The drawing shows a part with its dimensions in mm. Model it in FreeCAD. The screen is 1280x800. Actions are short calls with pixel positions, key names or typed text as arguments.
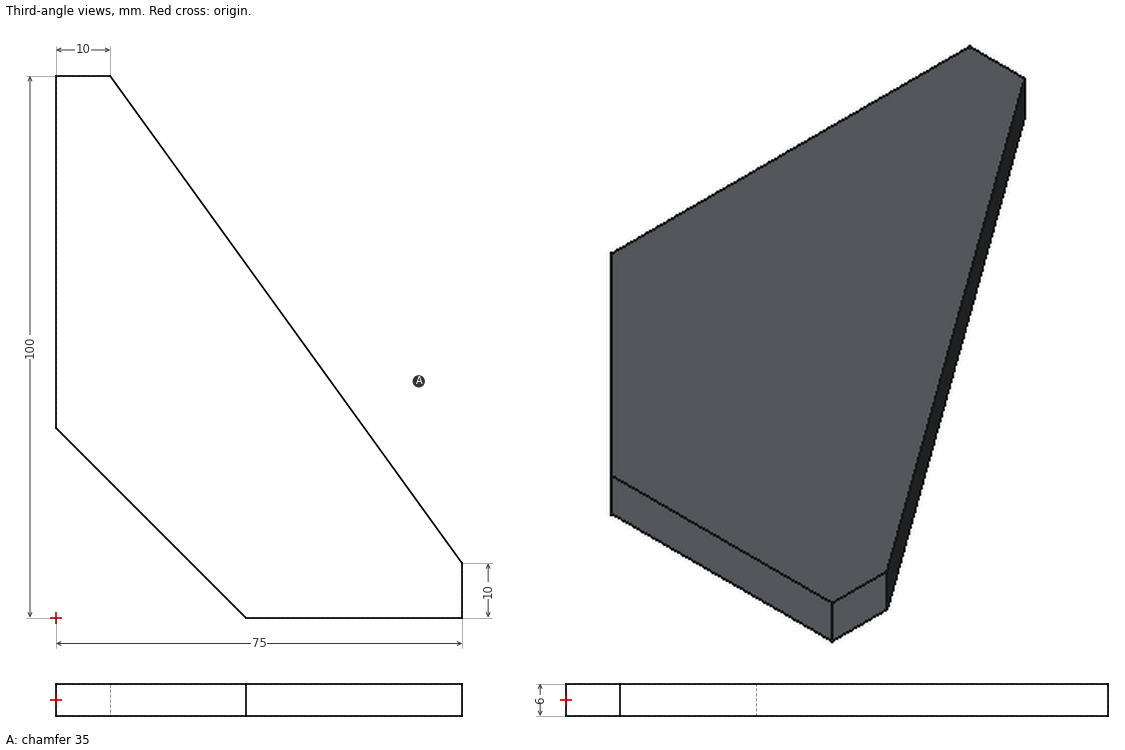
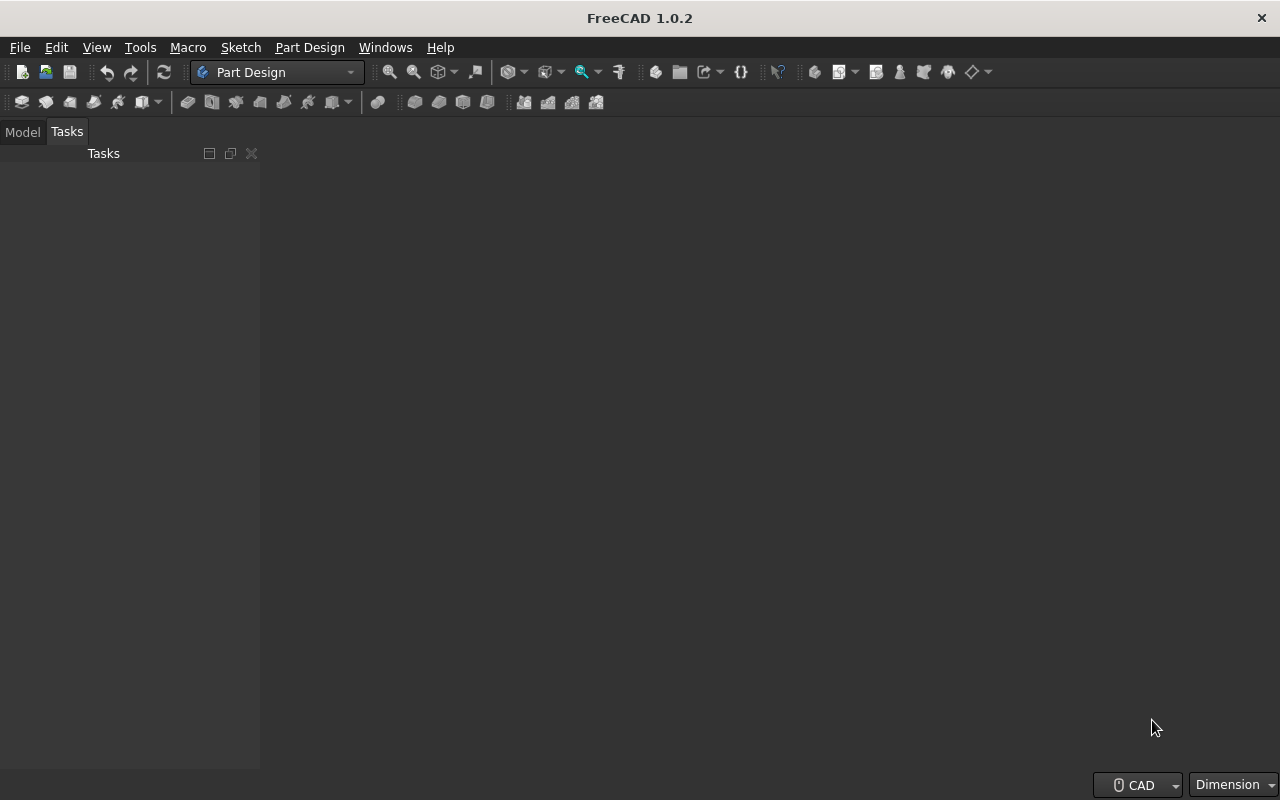
click(22, 72)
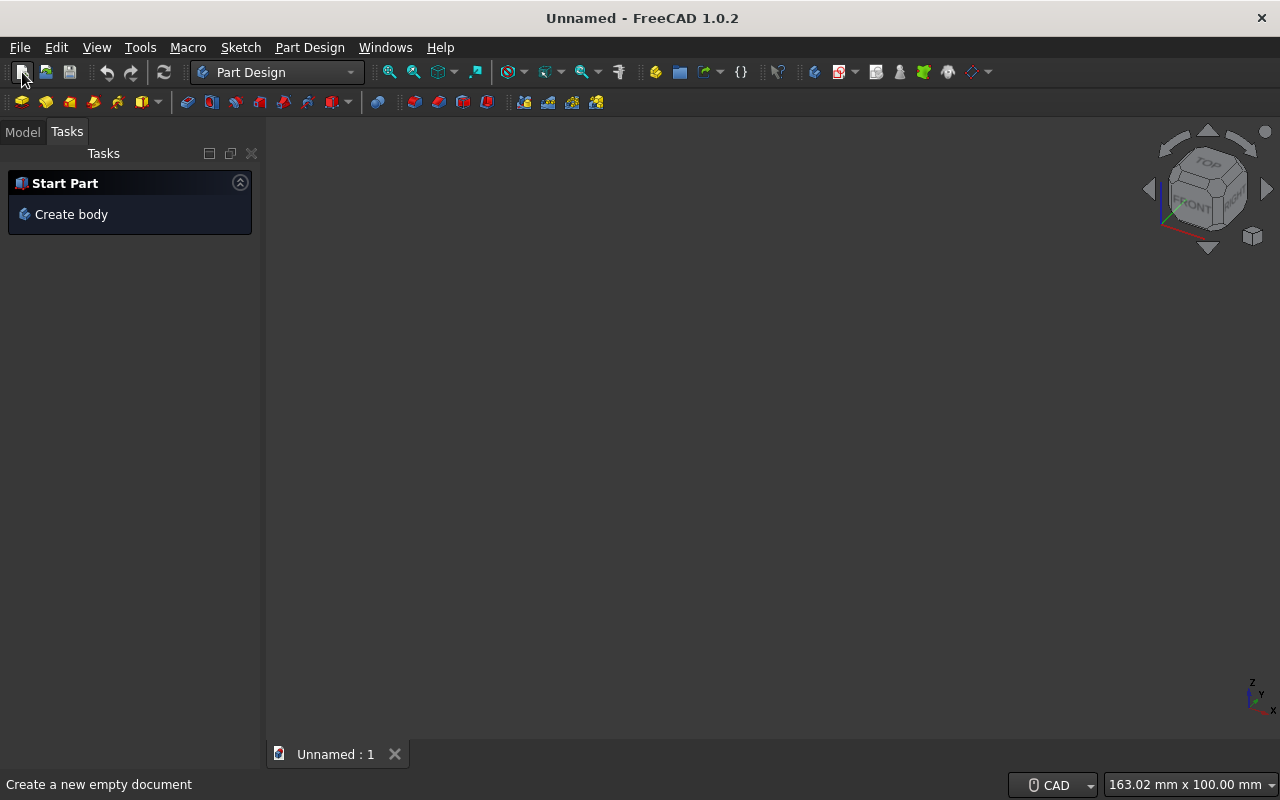
click(840, 72)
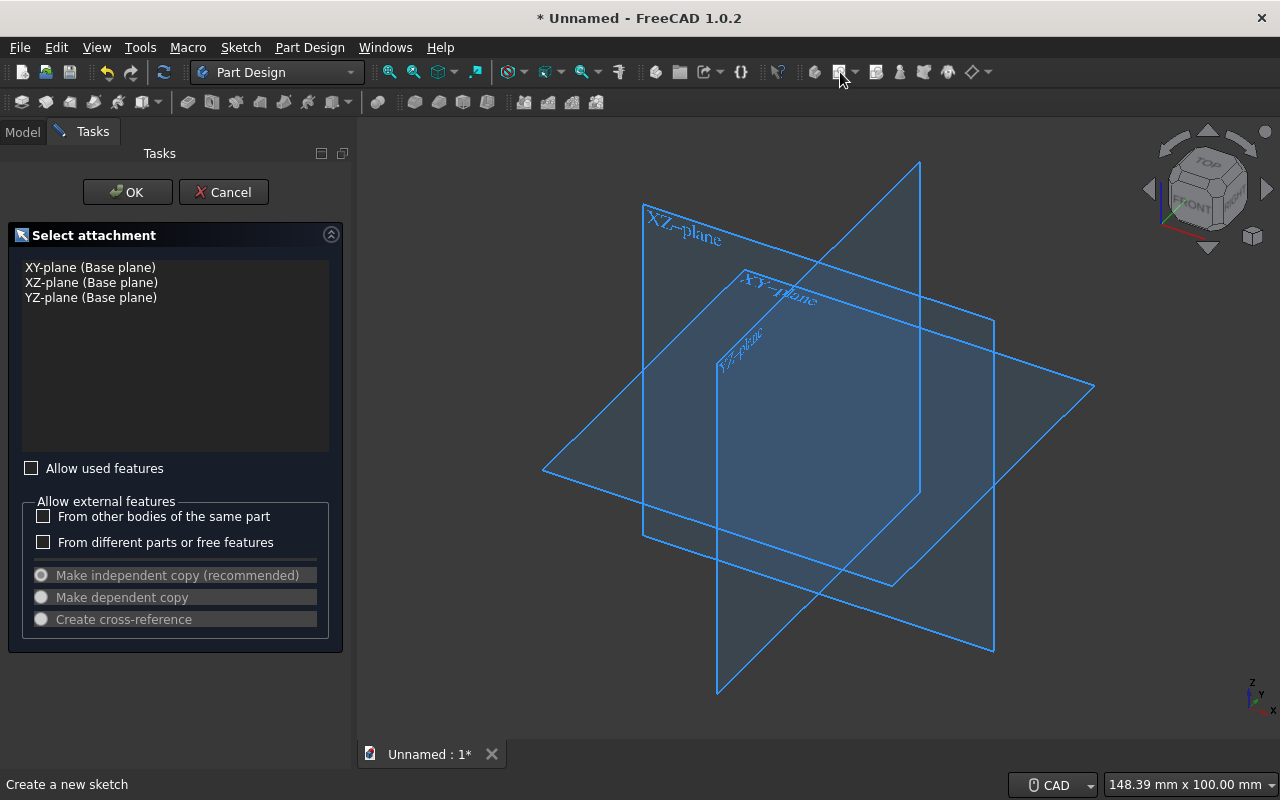
click(82, 268)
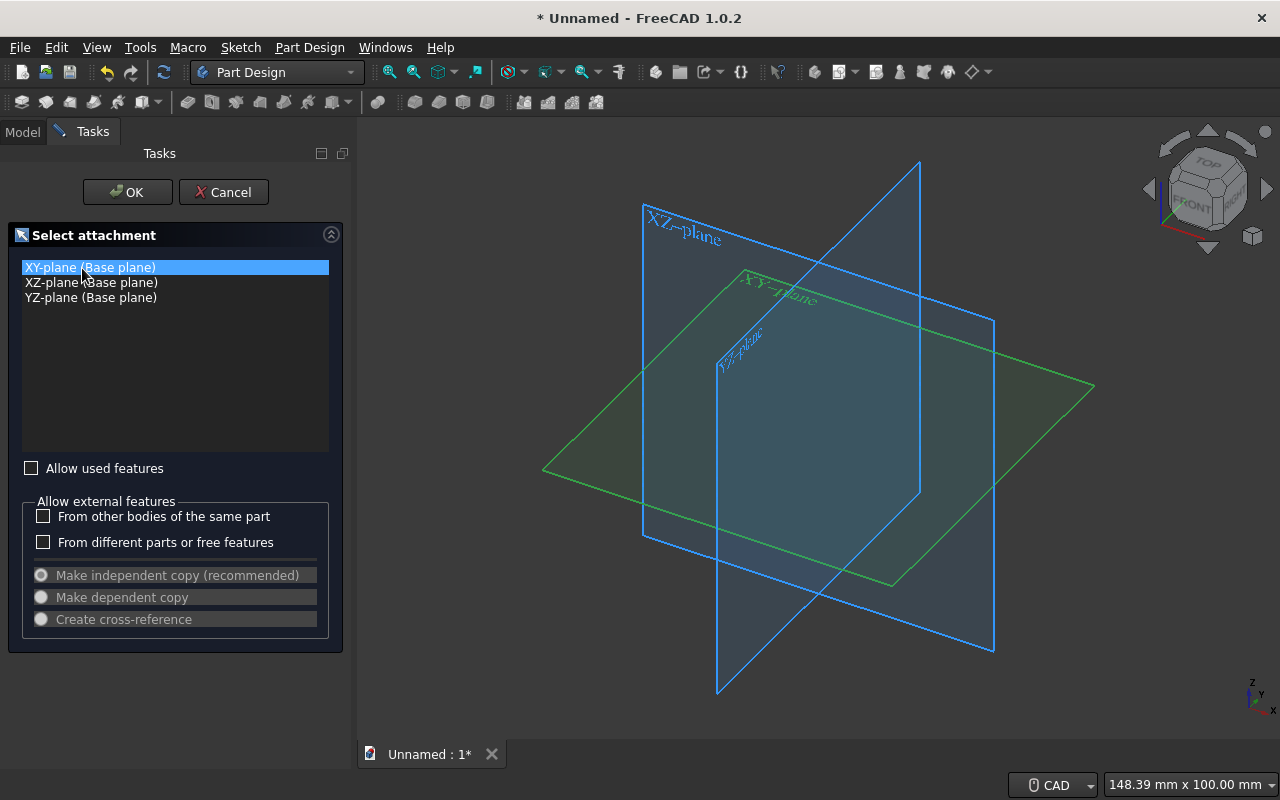
click(128, 192)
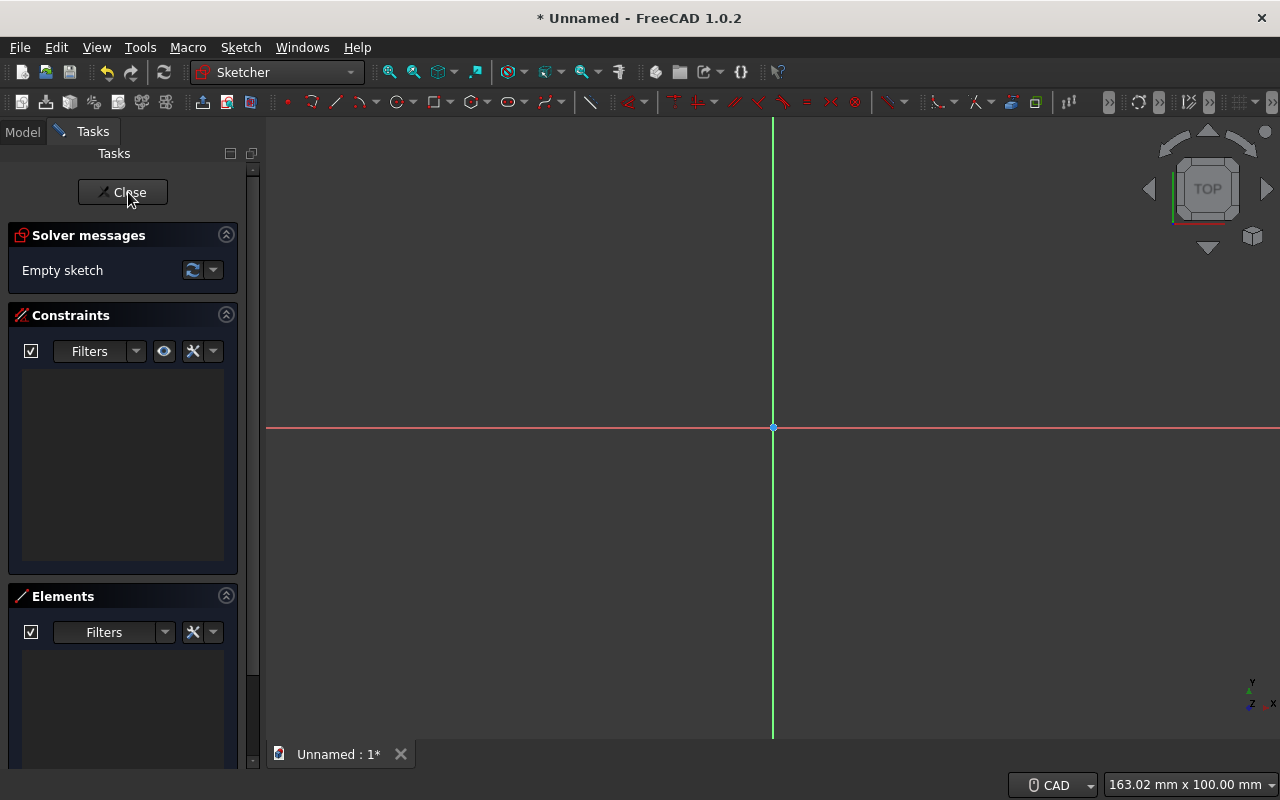
scroll(337, 711, down, 3)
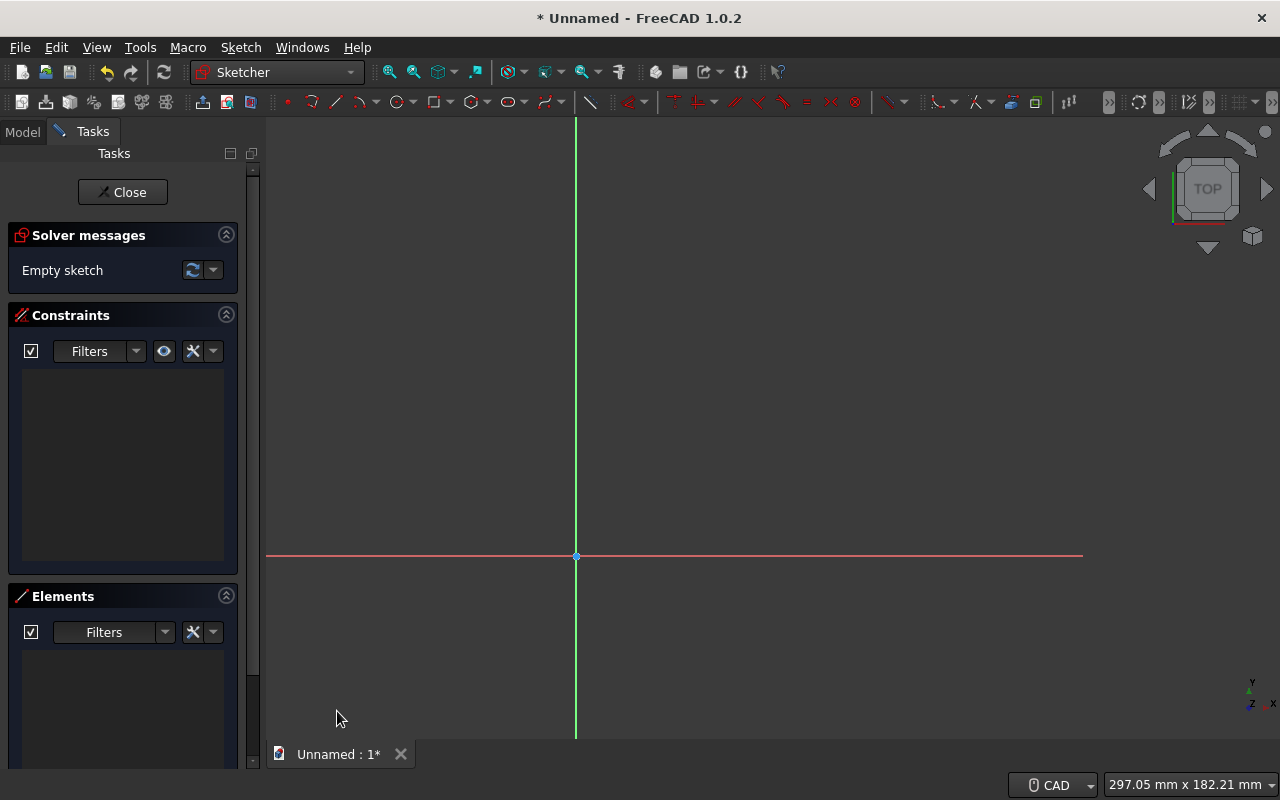
click(312, 102)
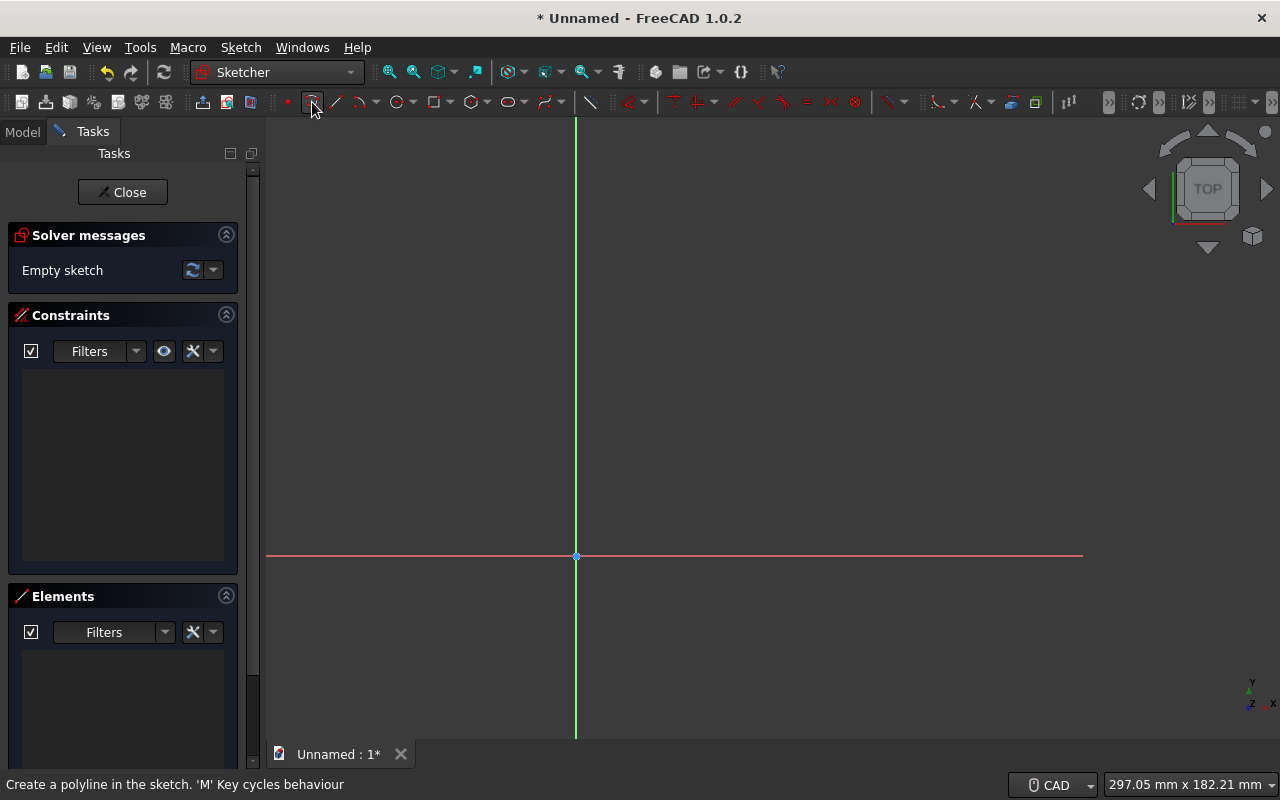
click(576, 556)
click(832, 547)
click(832, 522)
click(610, 215)
click(585, 215)
click(576, 556)
key(Escape)
key(Escape)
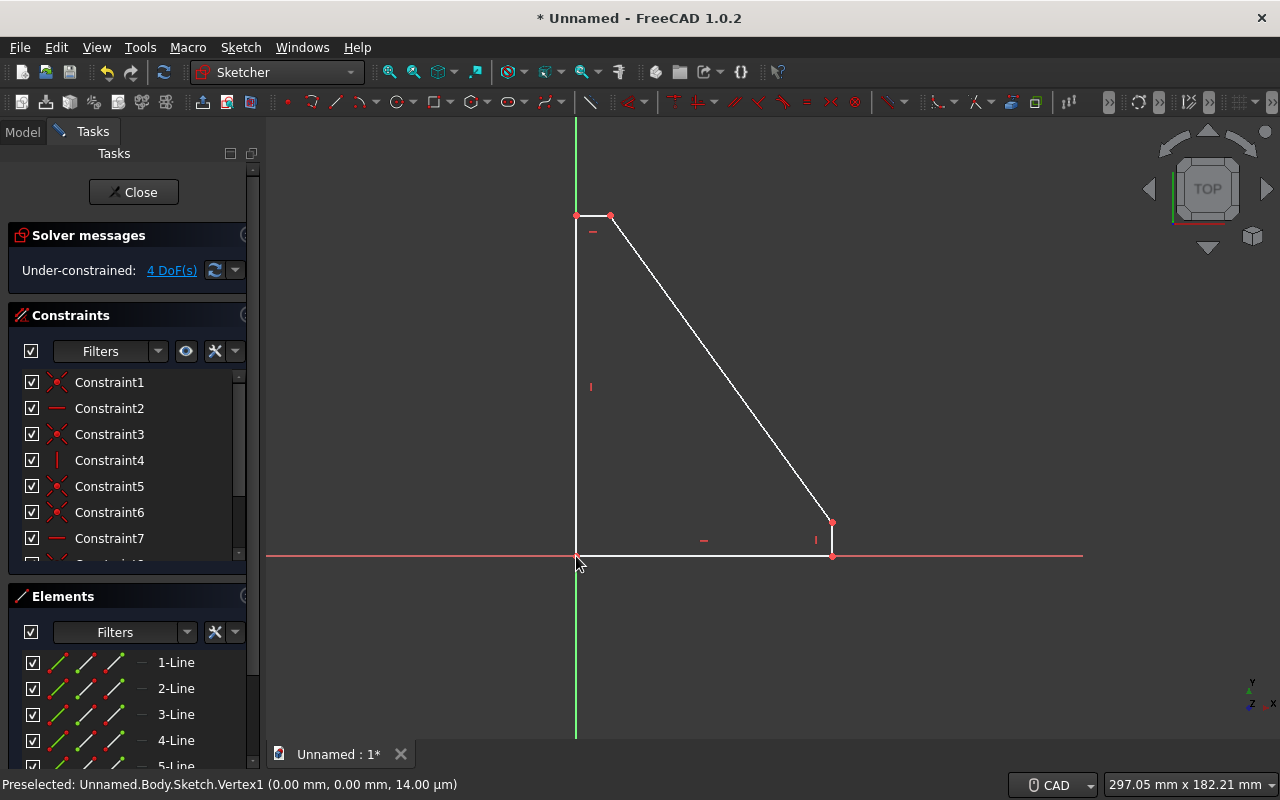
click(628, 102)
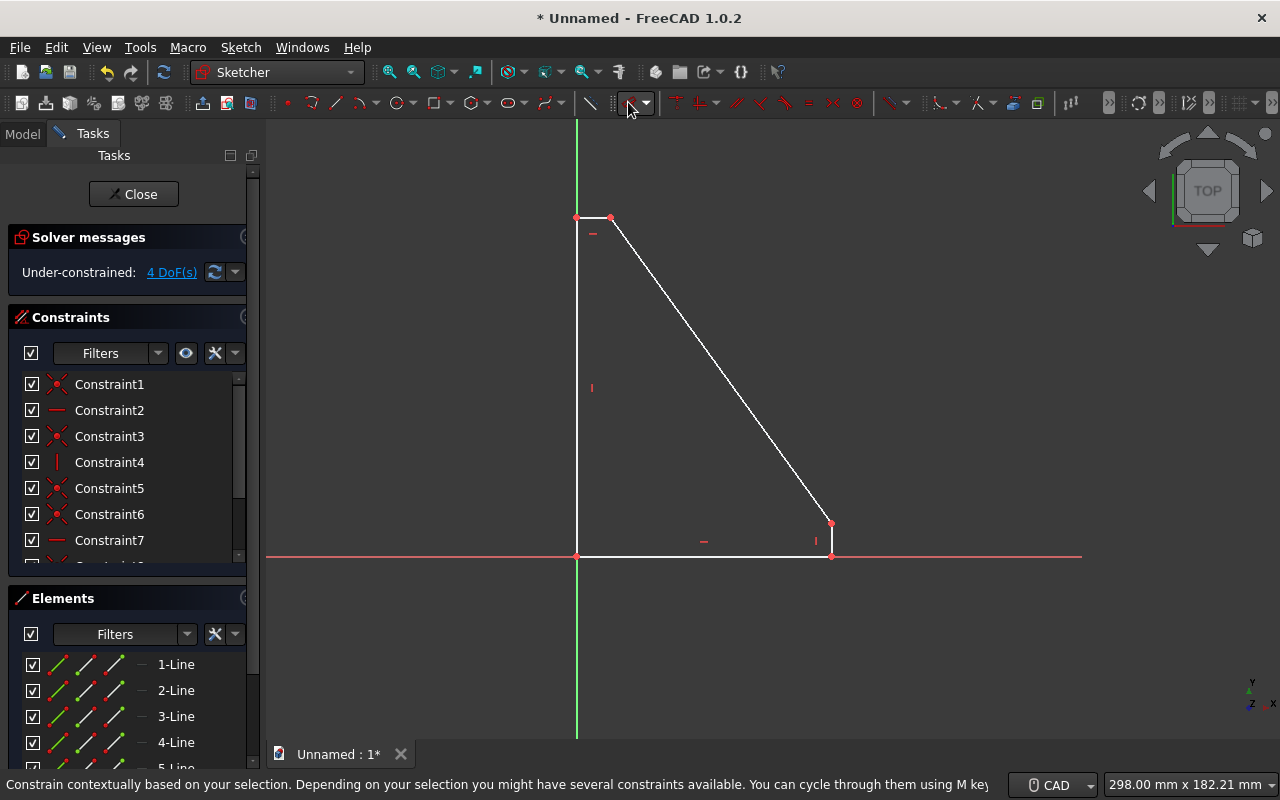
click(653, 557)
click(704, 591)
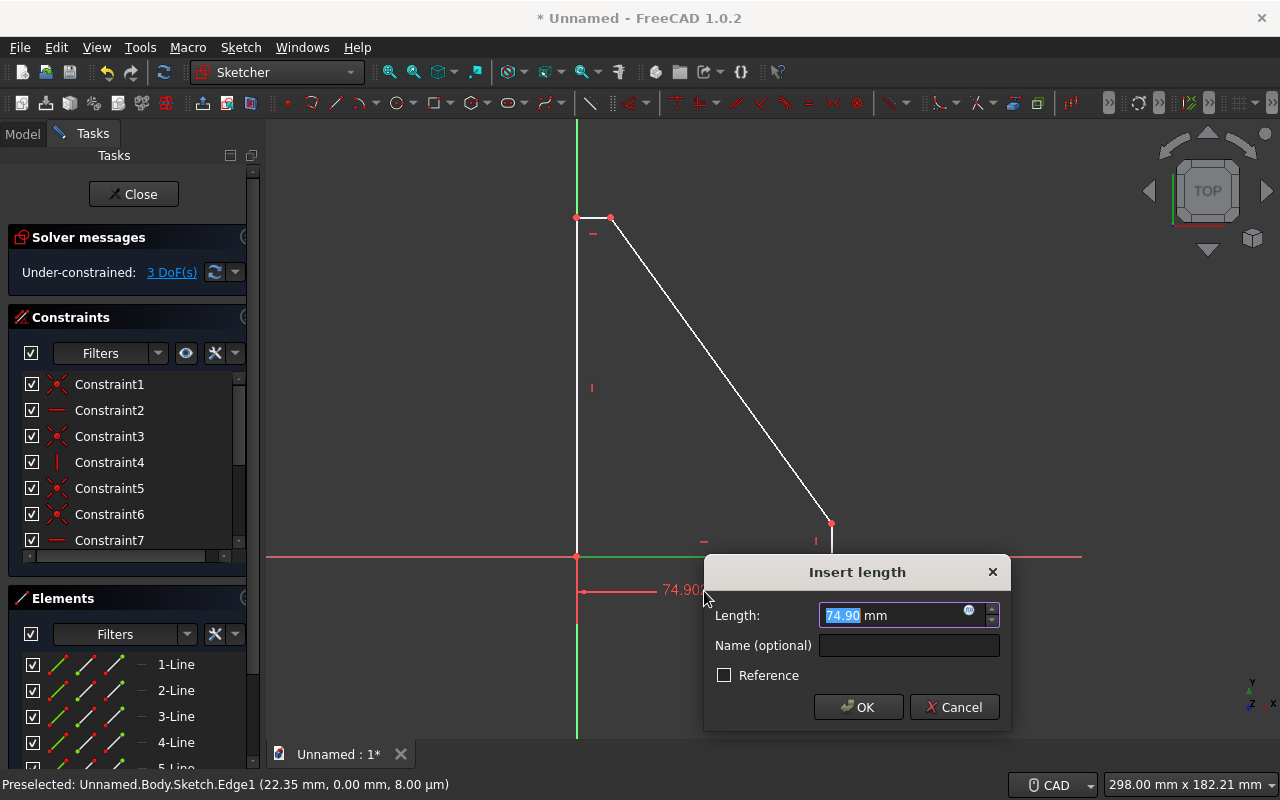
text(75)
key(Return)